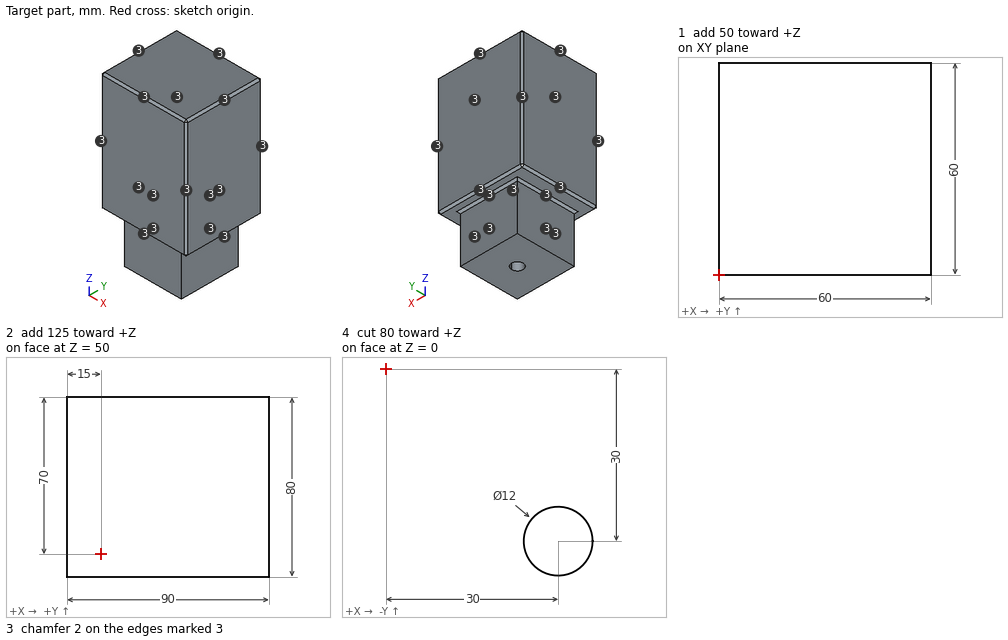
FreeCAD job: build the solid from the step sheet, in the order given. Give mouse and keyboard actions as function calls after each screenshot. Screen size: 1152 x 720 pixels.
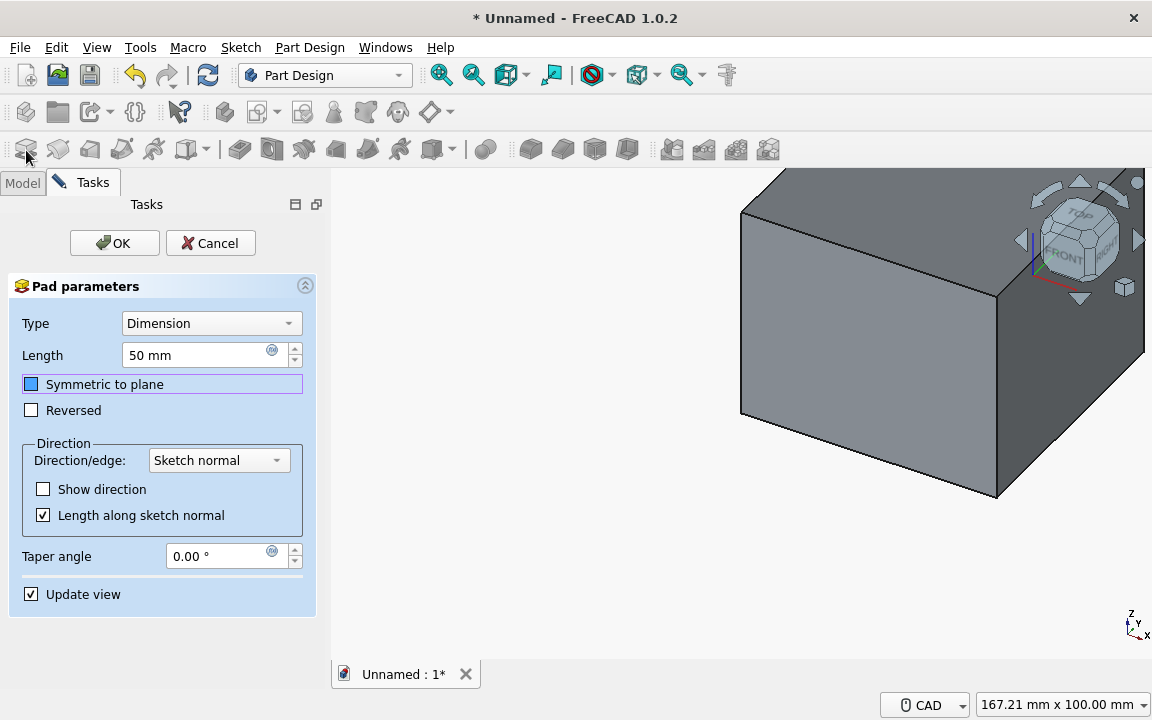
click(115, 243)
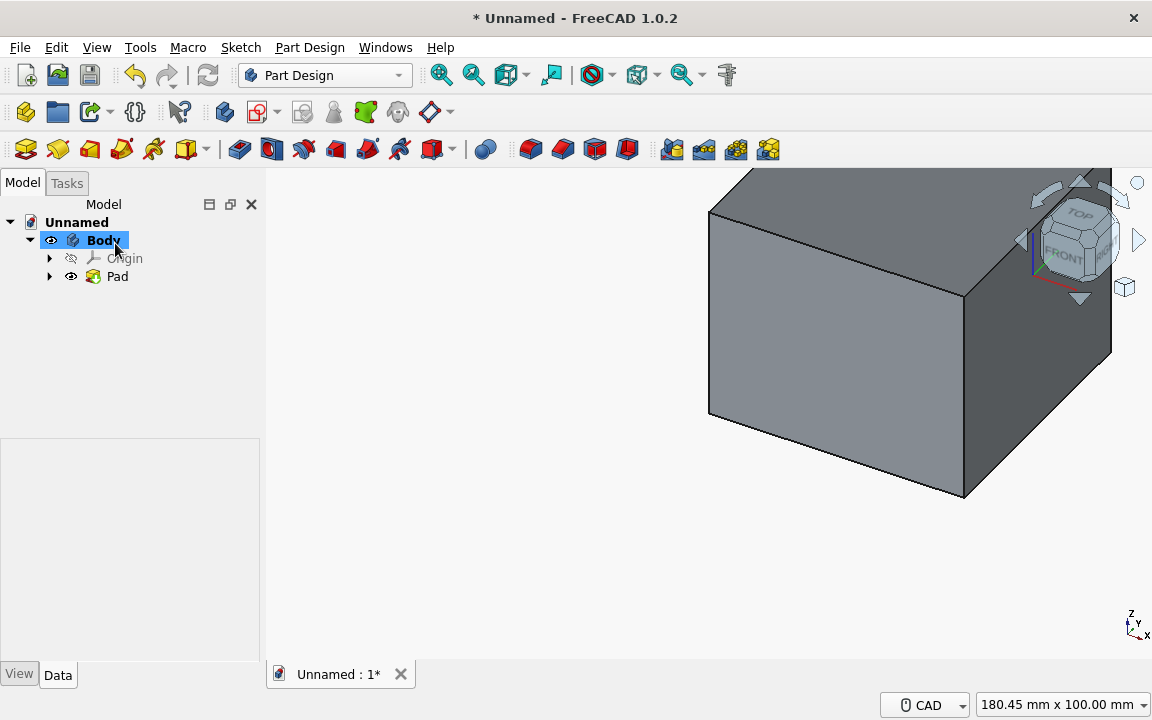
key(v)
key(f)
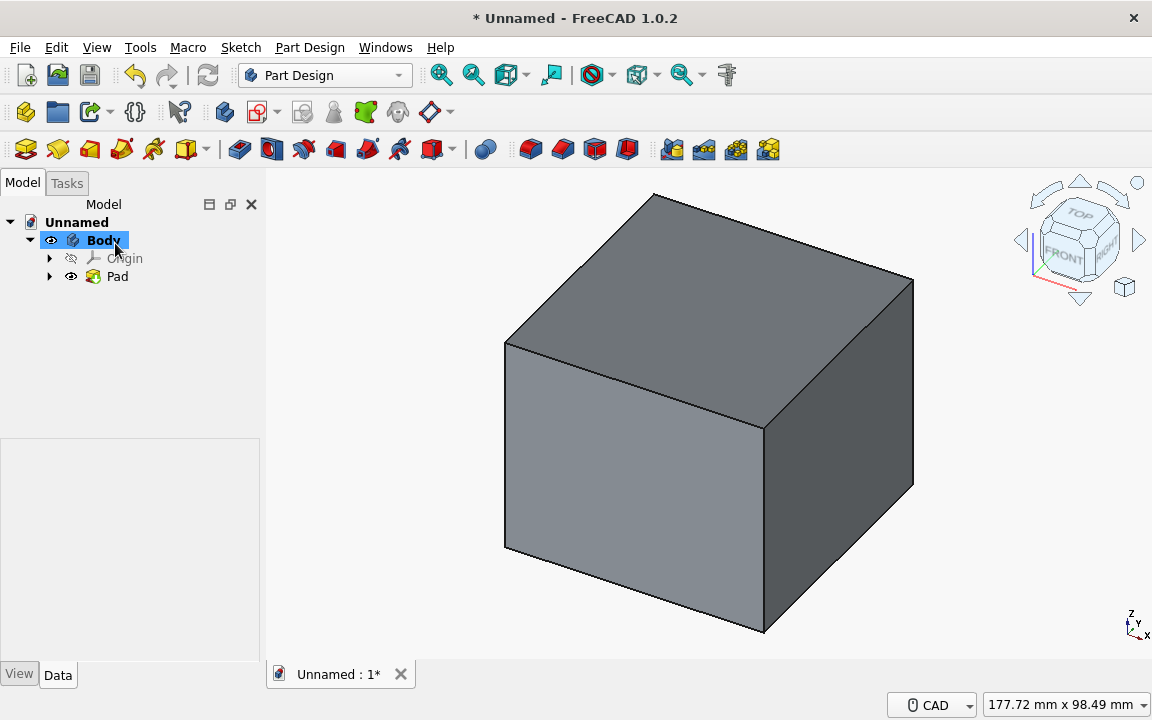
click(709, 310)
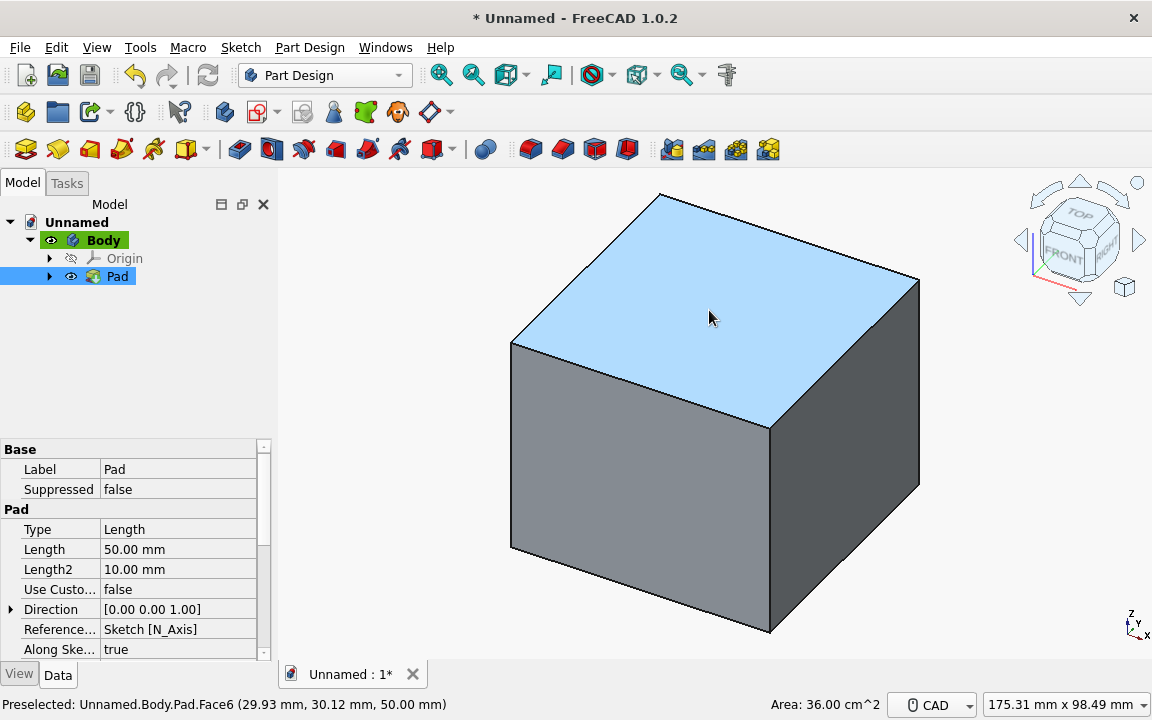
click(258, 112)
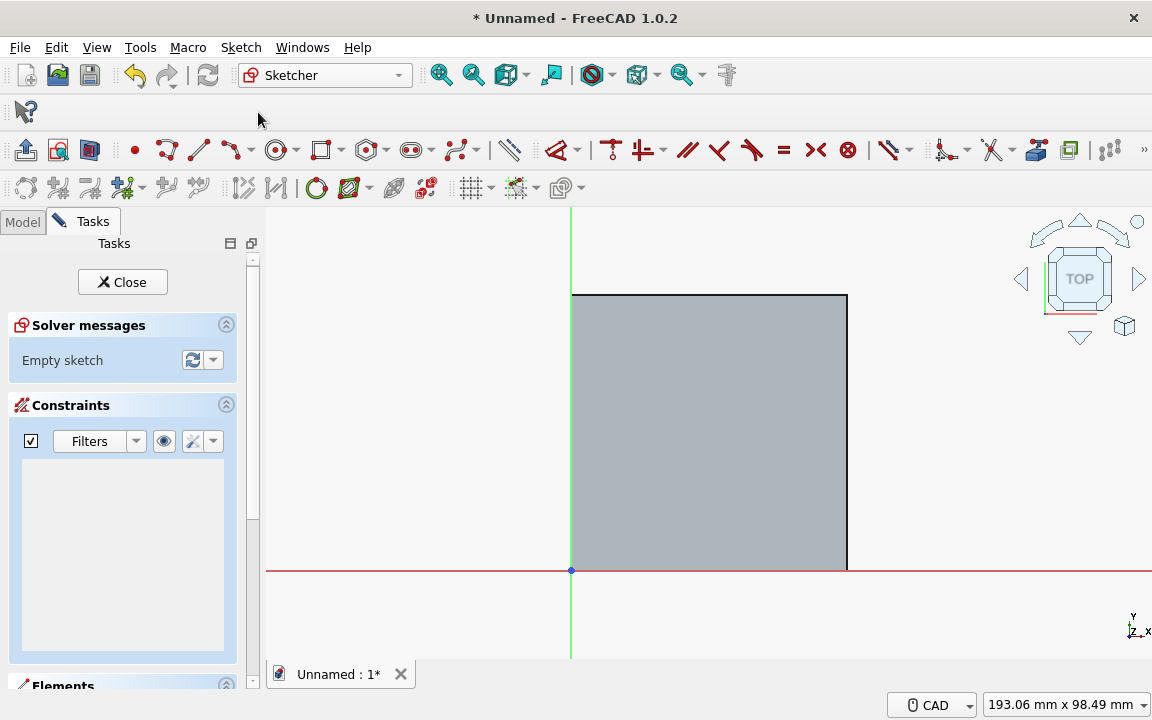
scroll(331, 433, down, 1)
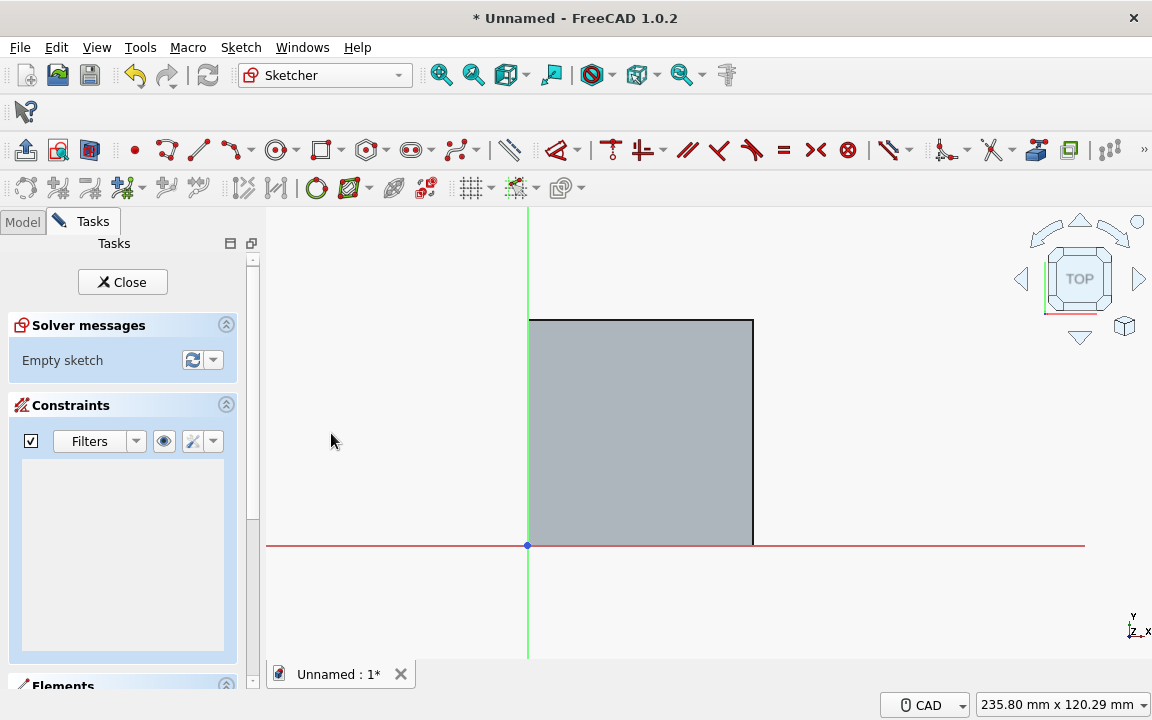
key(g)
key(r)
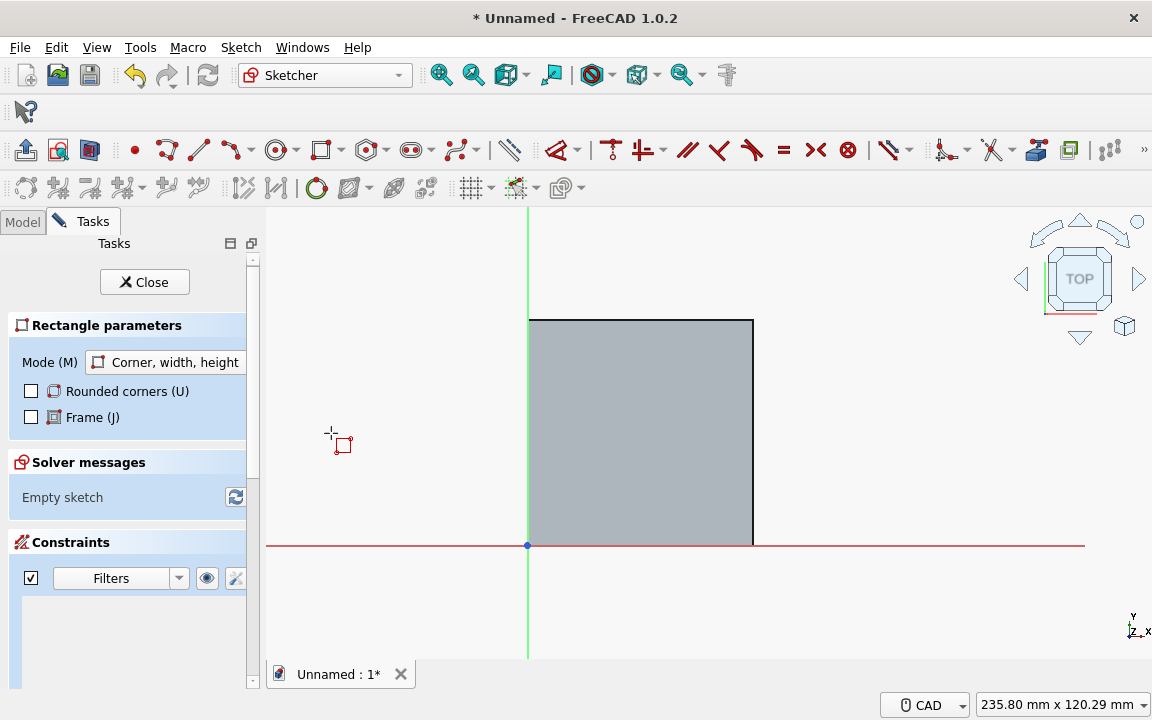
click(471, 283)
move(810, 583)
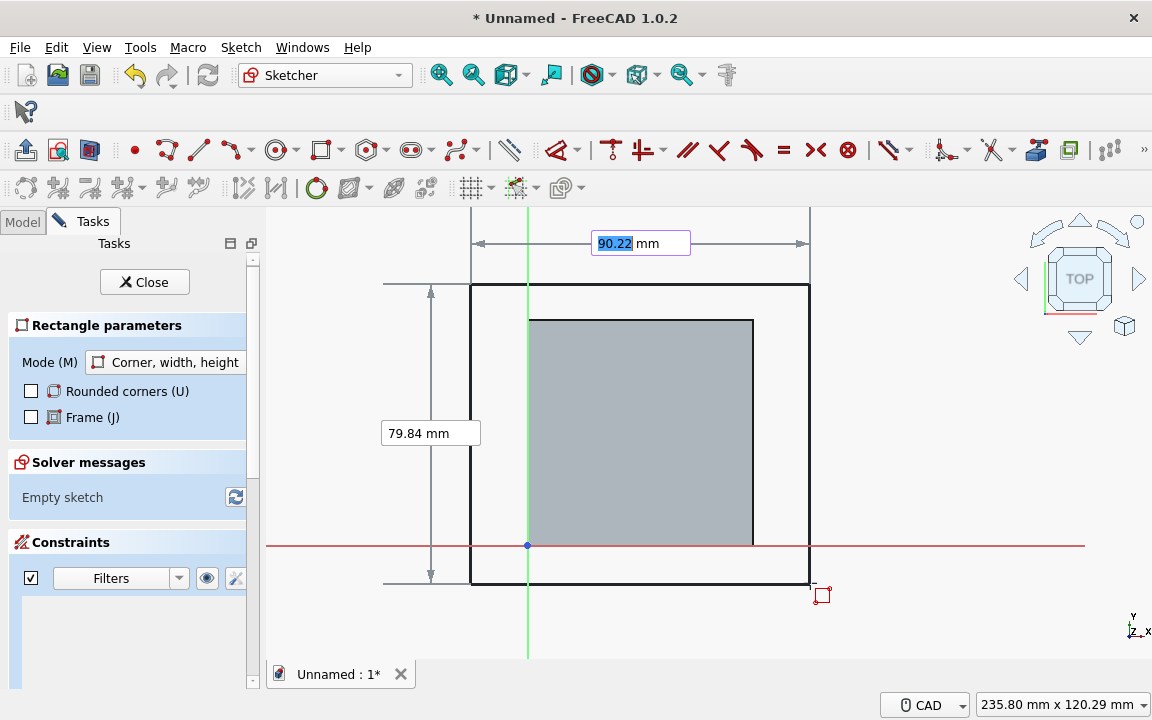
text(90)
key(Tab)
text(80)
key(Return)
key(Escape)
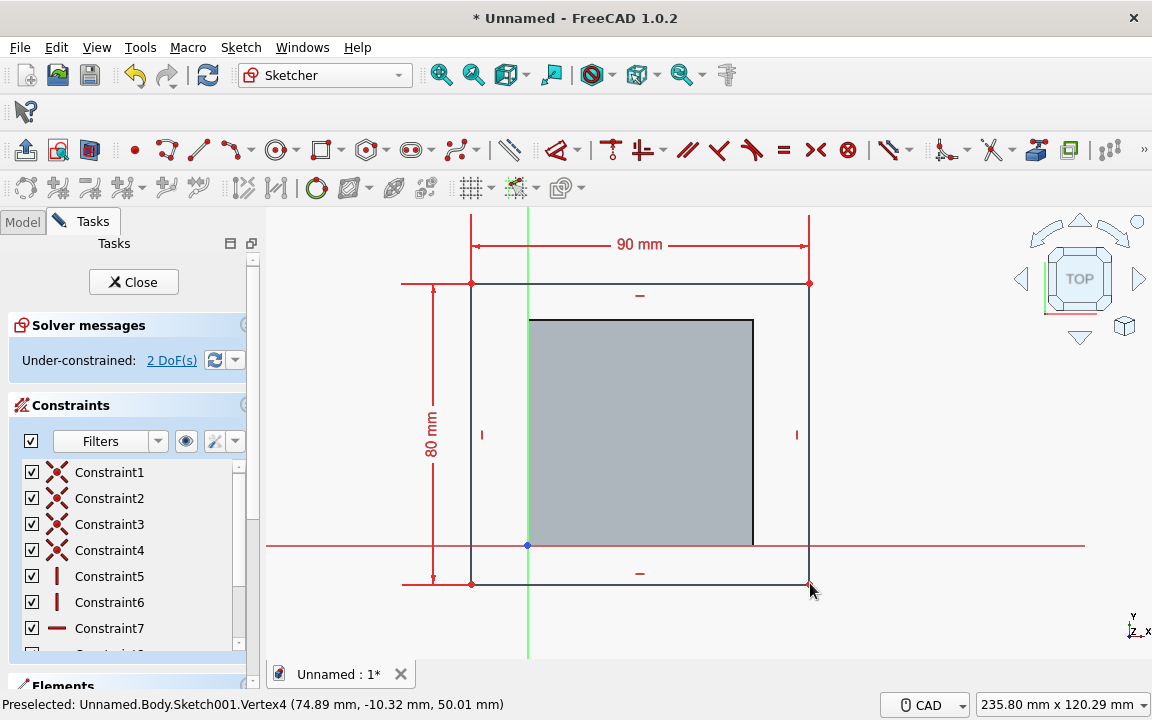
click(471, 284)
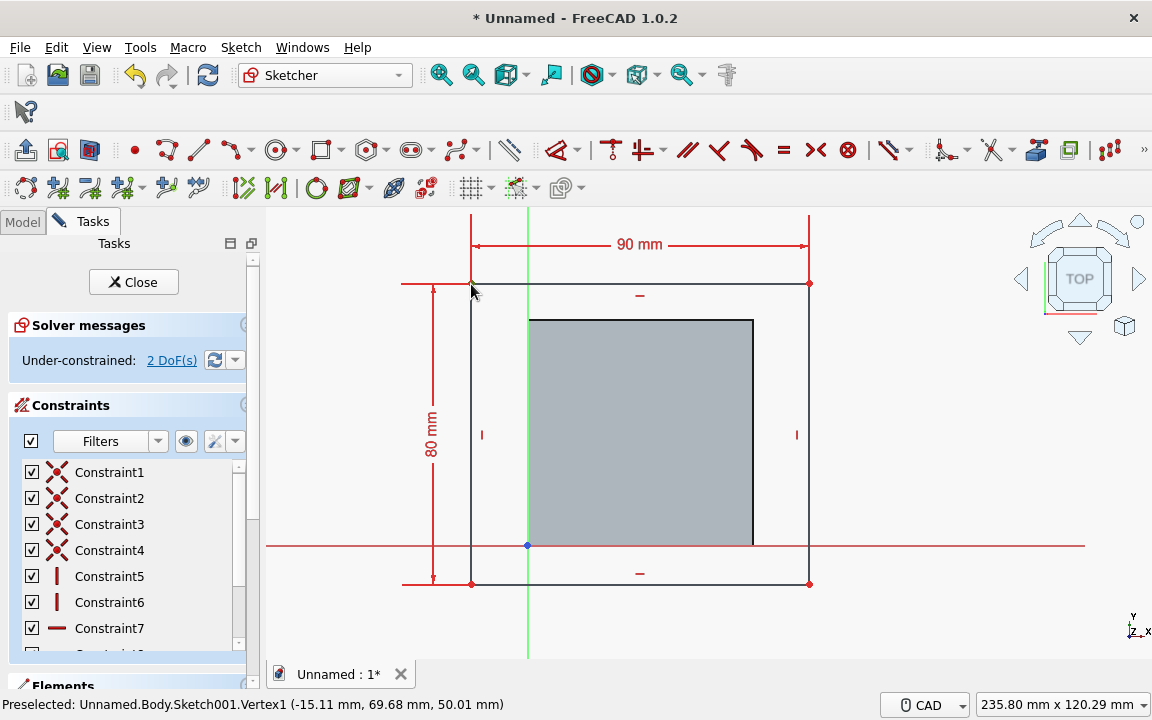
key(l)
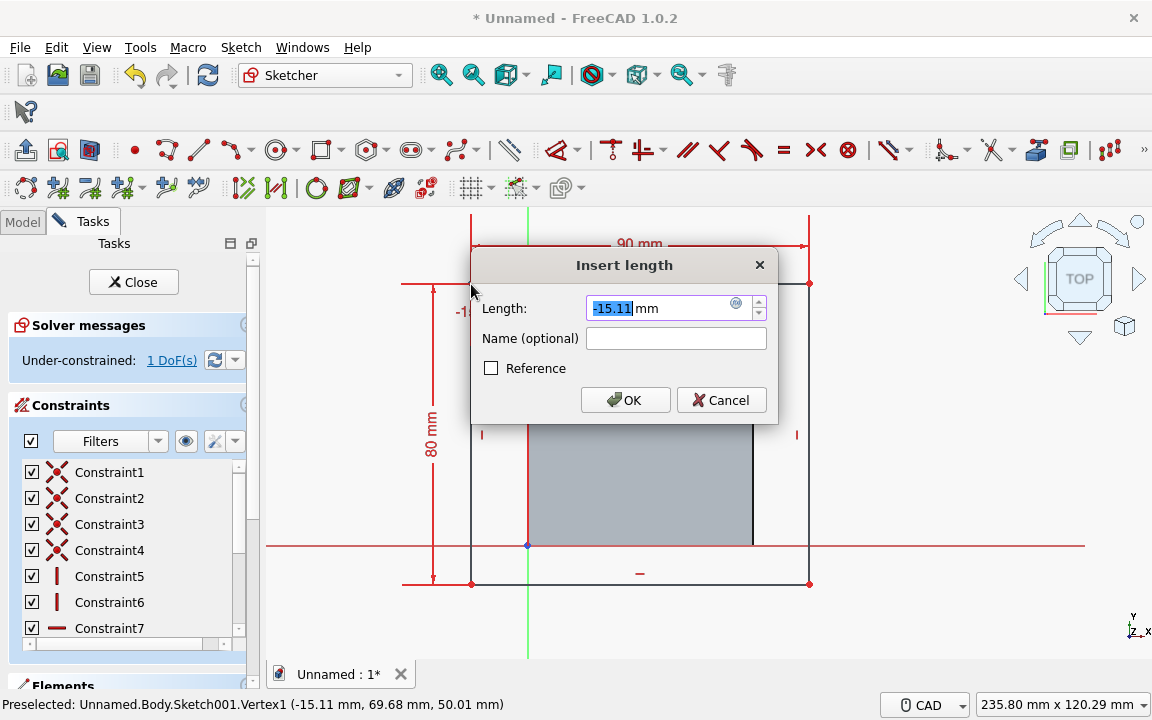
text(-15)
key(Return)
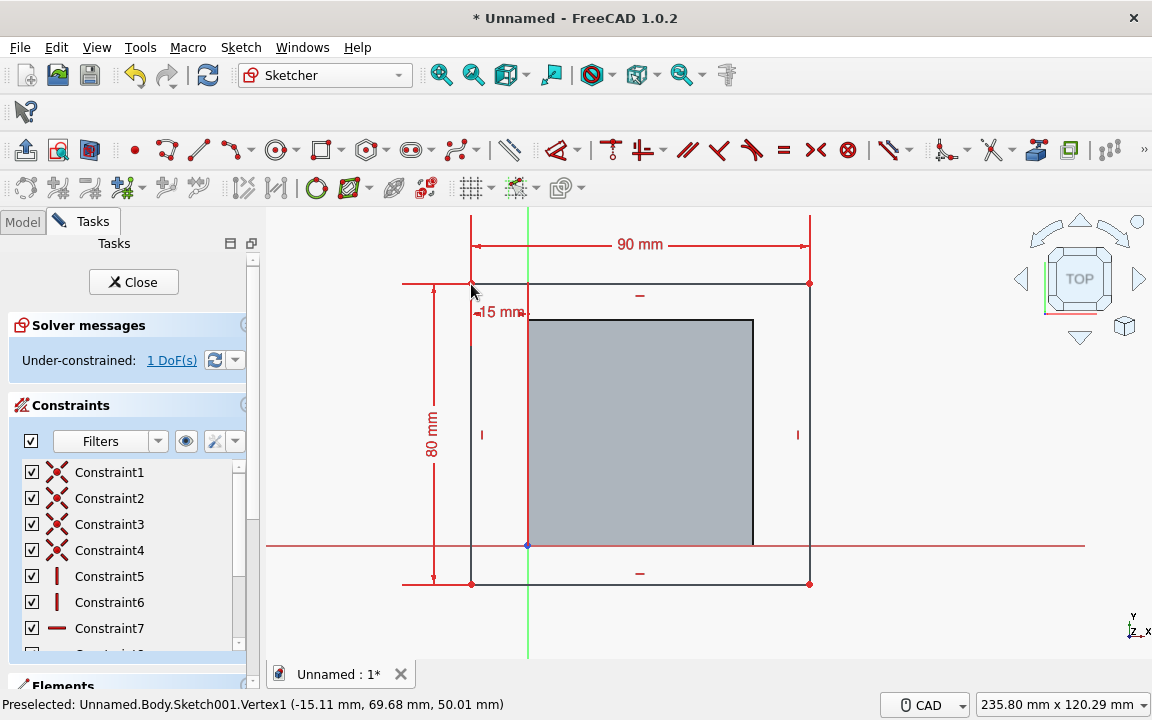
click(471, 284)